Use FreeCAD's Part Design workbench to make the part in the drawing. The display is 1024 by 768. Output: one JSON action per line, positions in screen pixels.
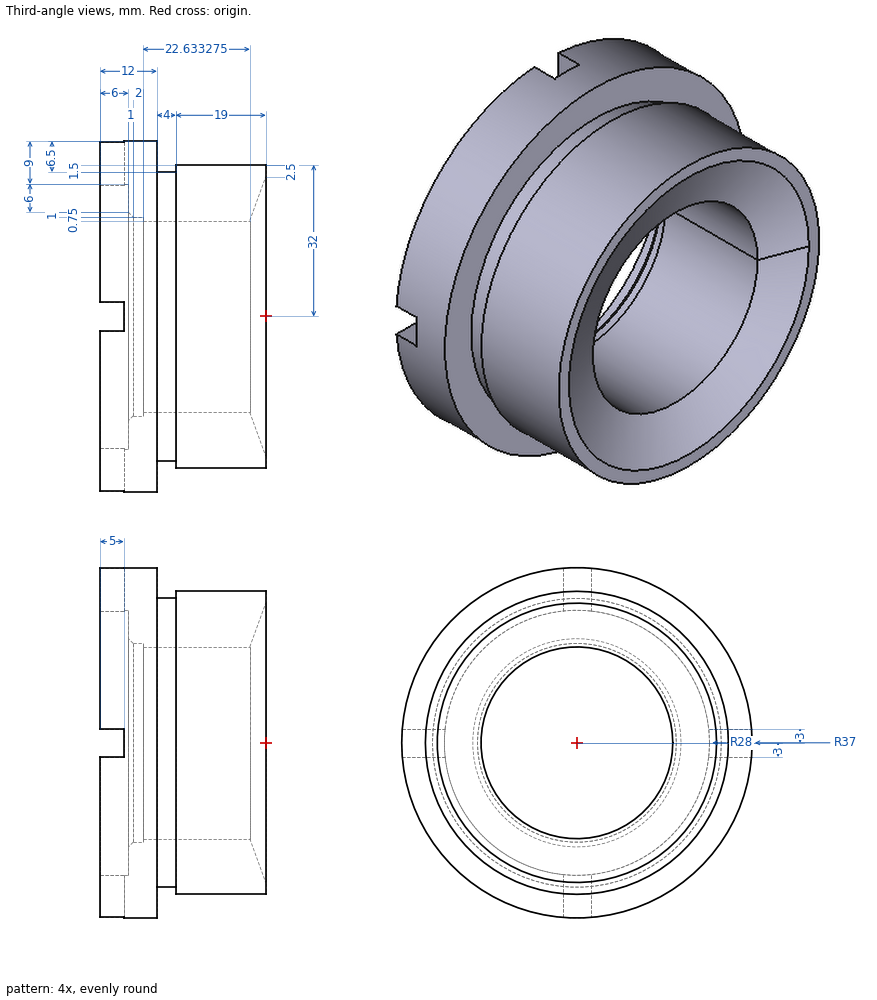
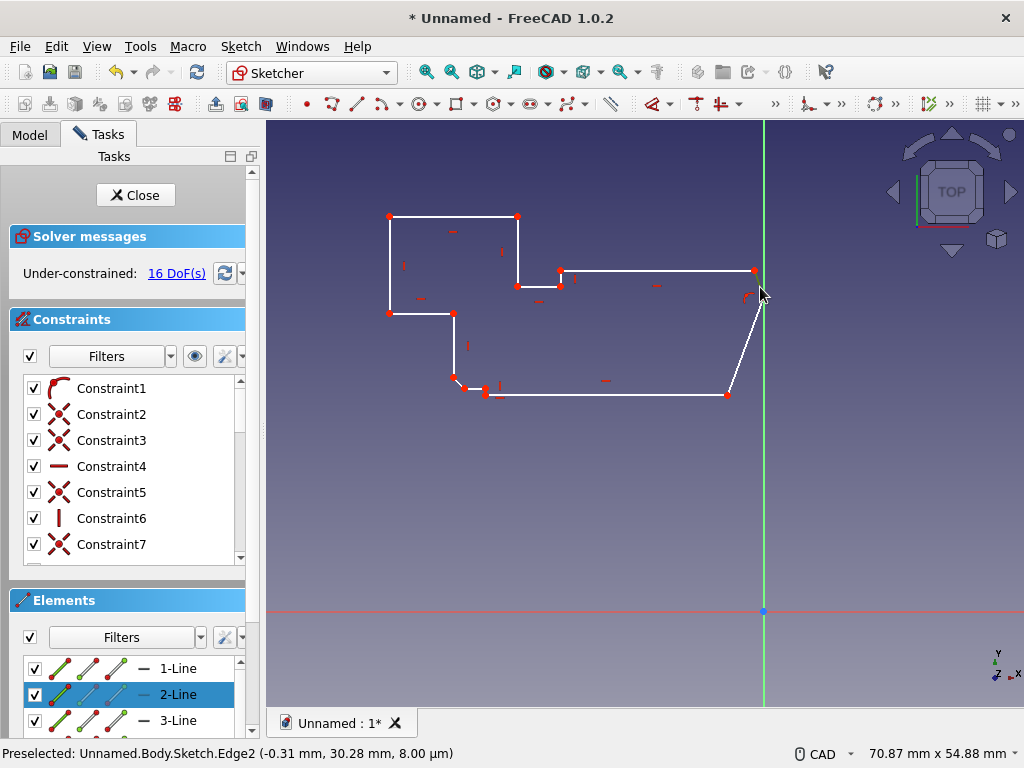
{"action": "left_click", "coordinate": [738, 104]}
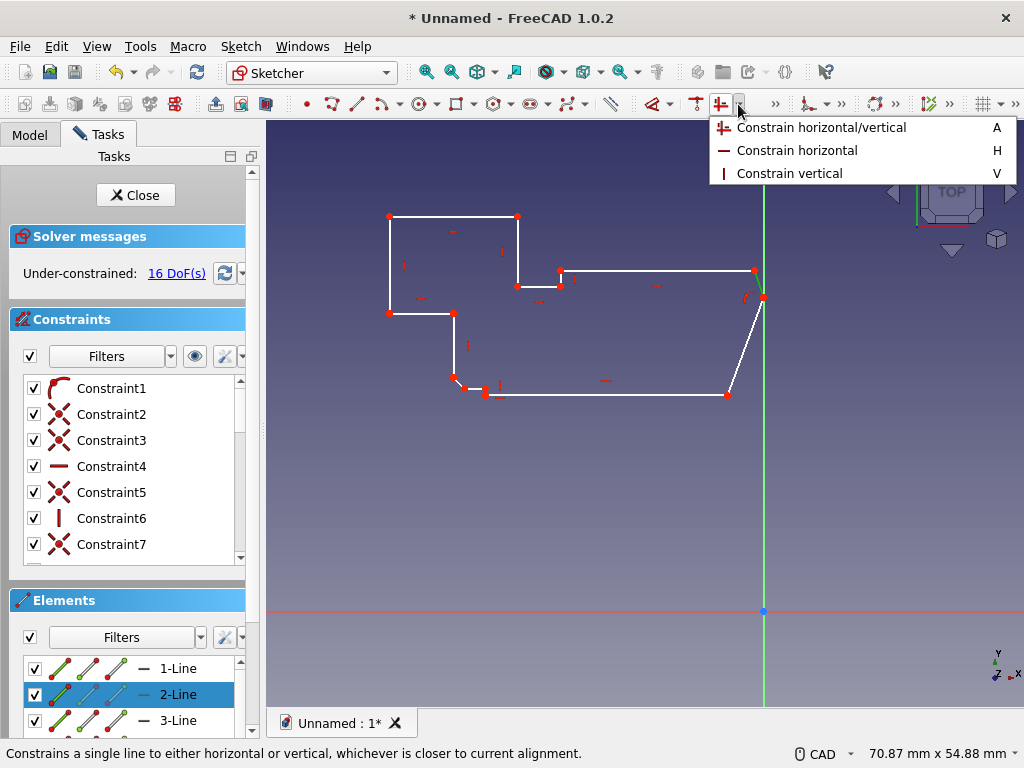
{"action": "left_click", "coordinate": [863, 174]}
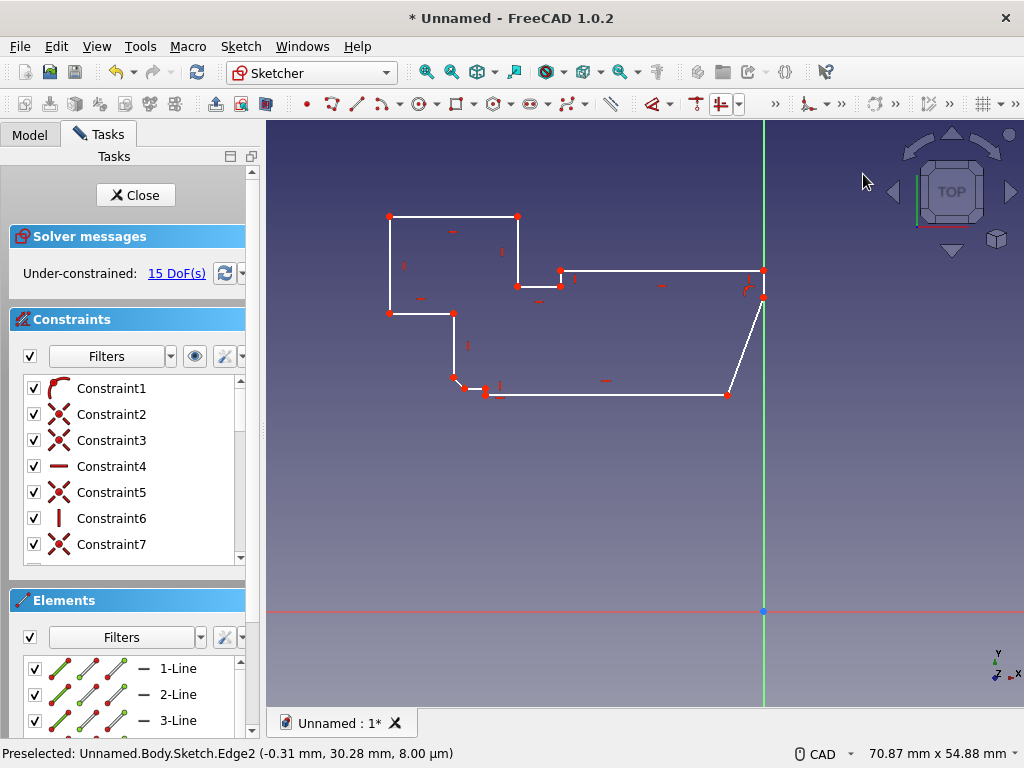
{"action": "left_click", "coordinate": [652, 104]}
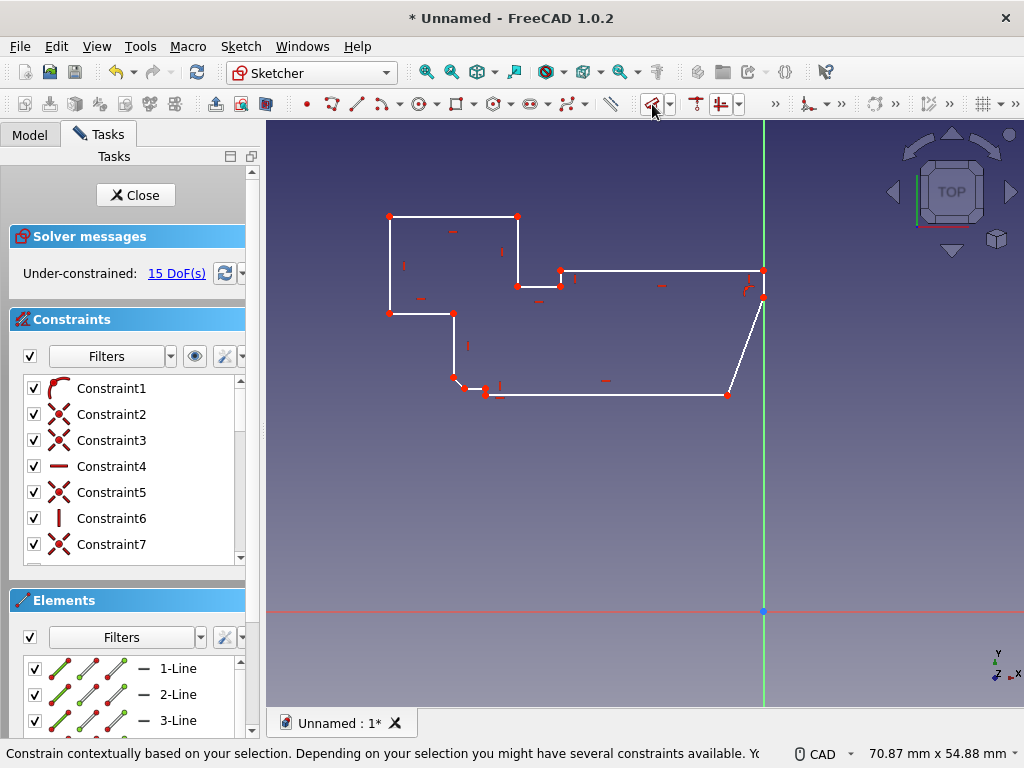
{"action": "left_click", "coordinate": [548, 287]}
{"action": "left_click", "coordinate": [539, 253]}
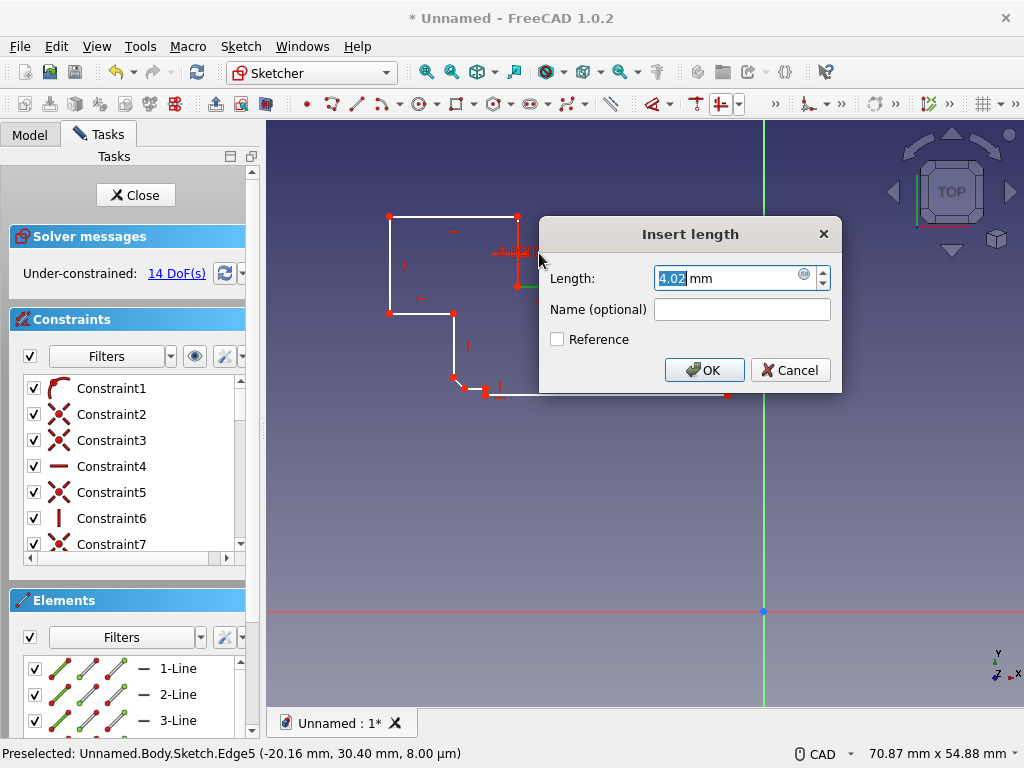
{"action": "type", "text": "4"}
{"action": "key", "text": "Return"}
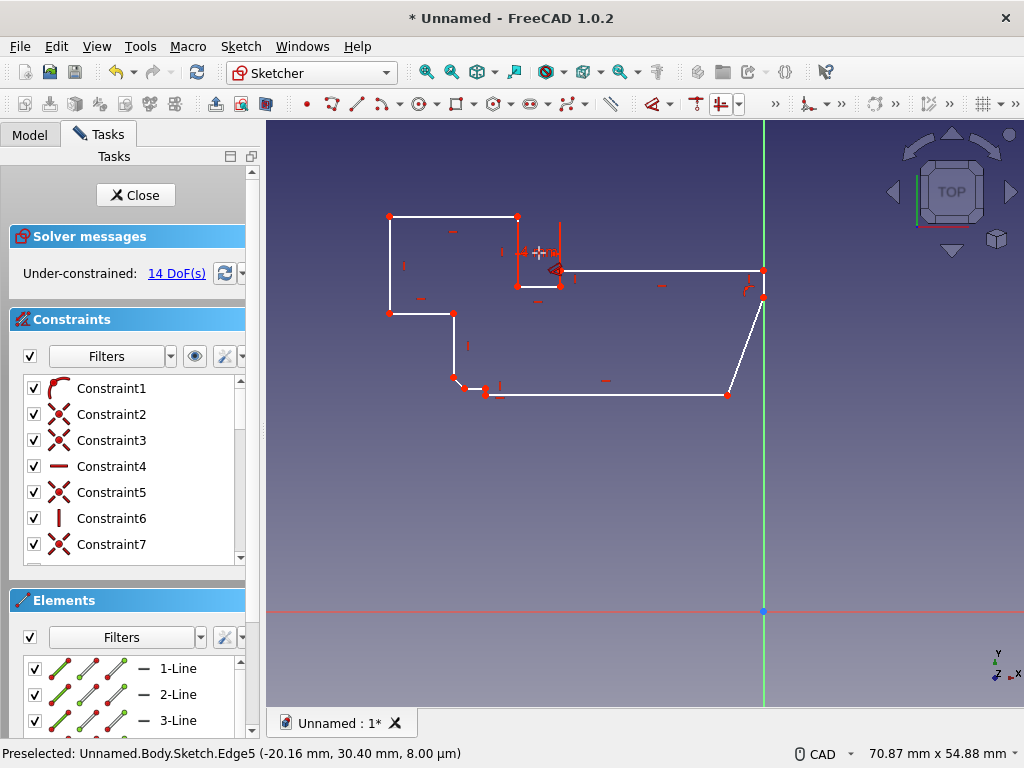
{"action": "left_click", "coordinate": [390, 246]}
{"action": "left_click", "coordinate": [356, 265]}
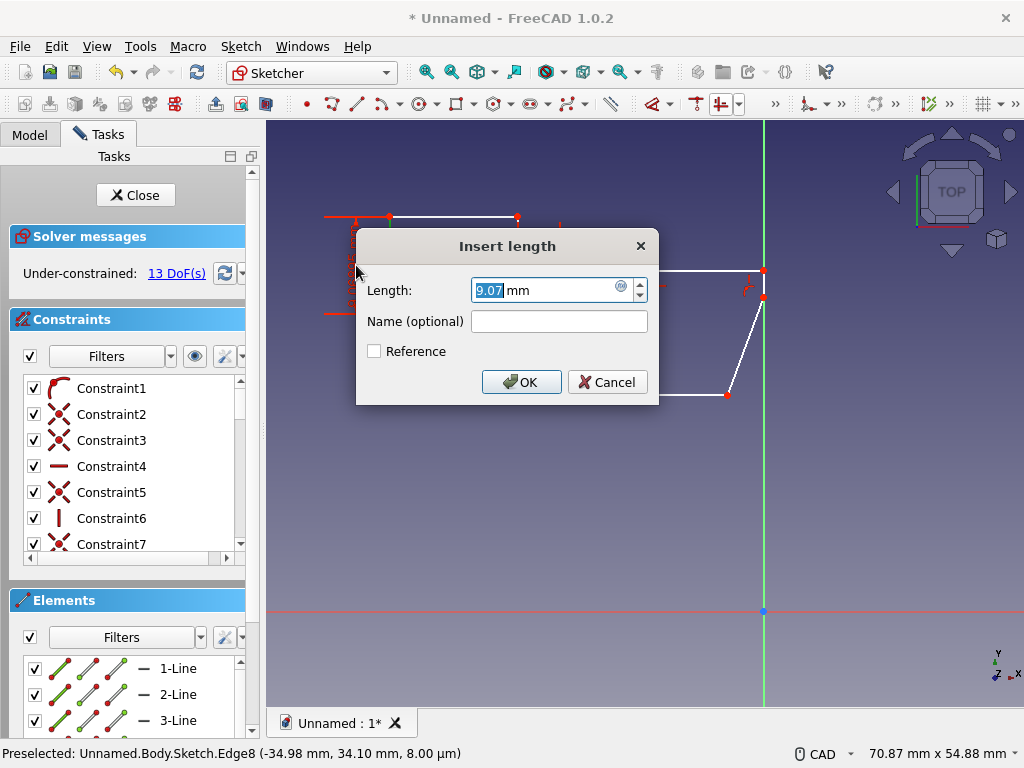
{"action": "type", "text": "9"}
{"action": "key", "text": "Return"}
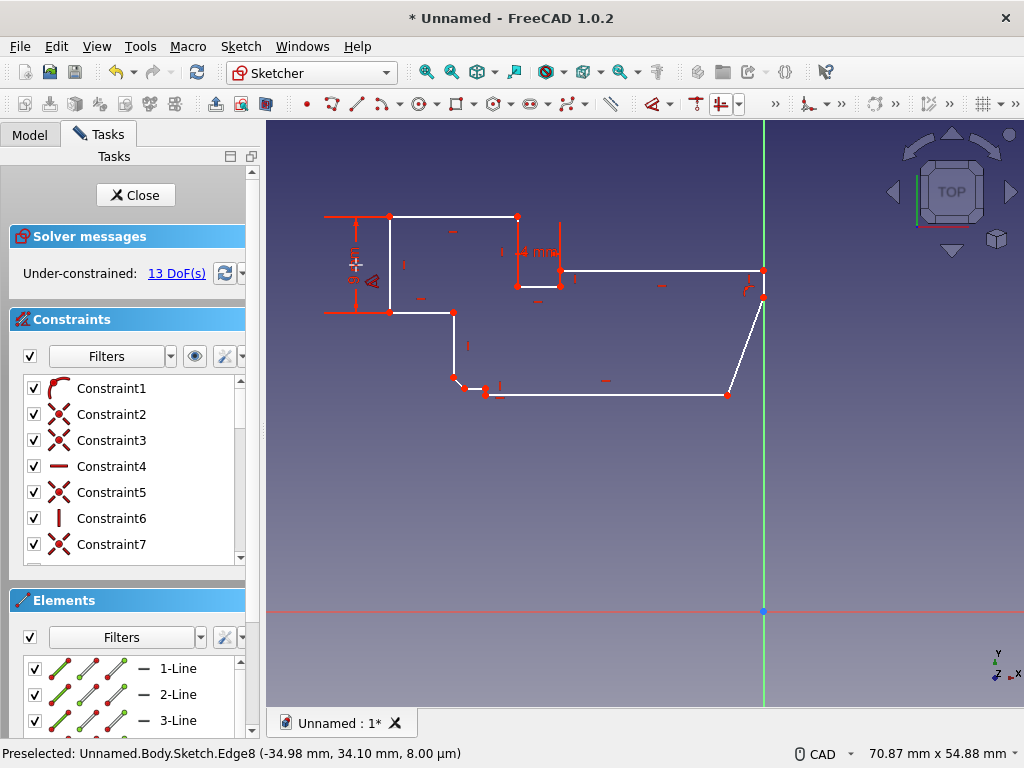
{"action": "left_click", "coordinate": [409, 313]}
{"action": "left_click", "coordinate": [436, 279]}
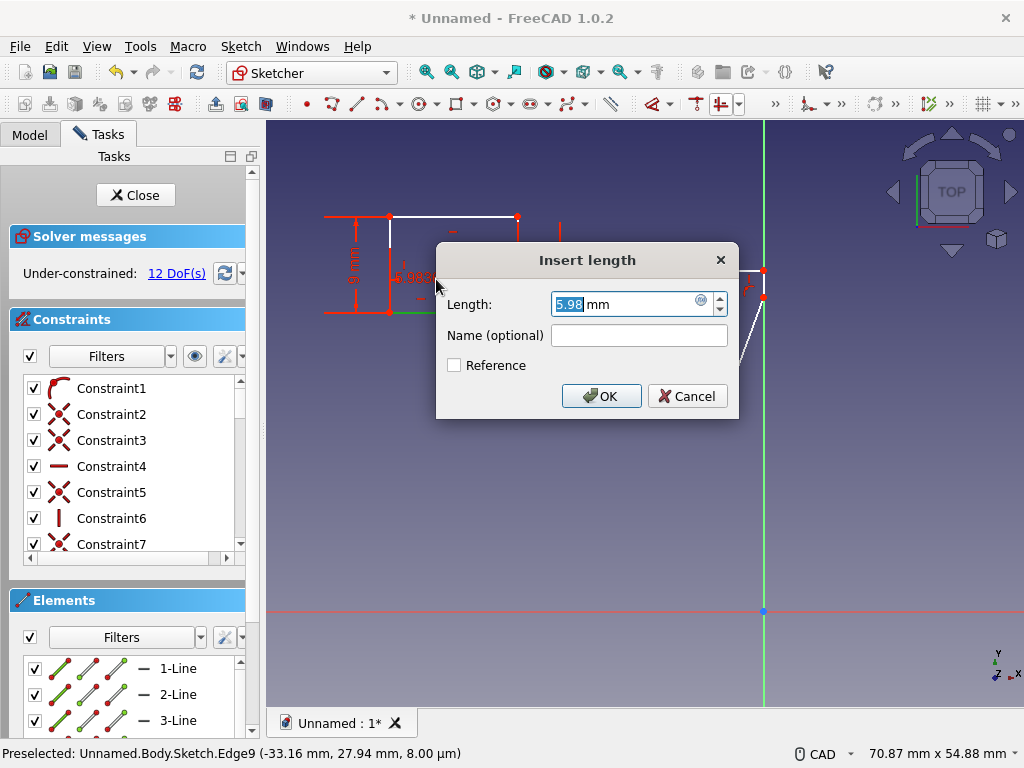
{"action": "type", "text": "6"}
{"action": "key", "text": "Return"}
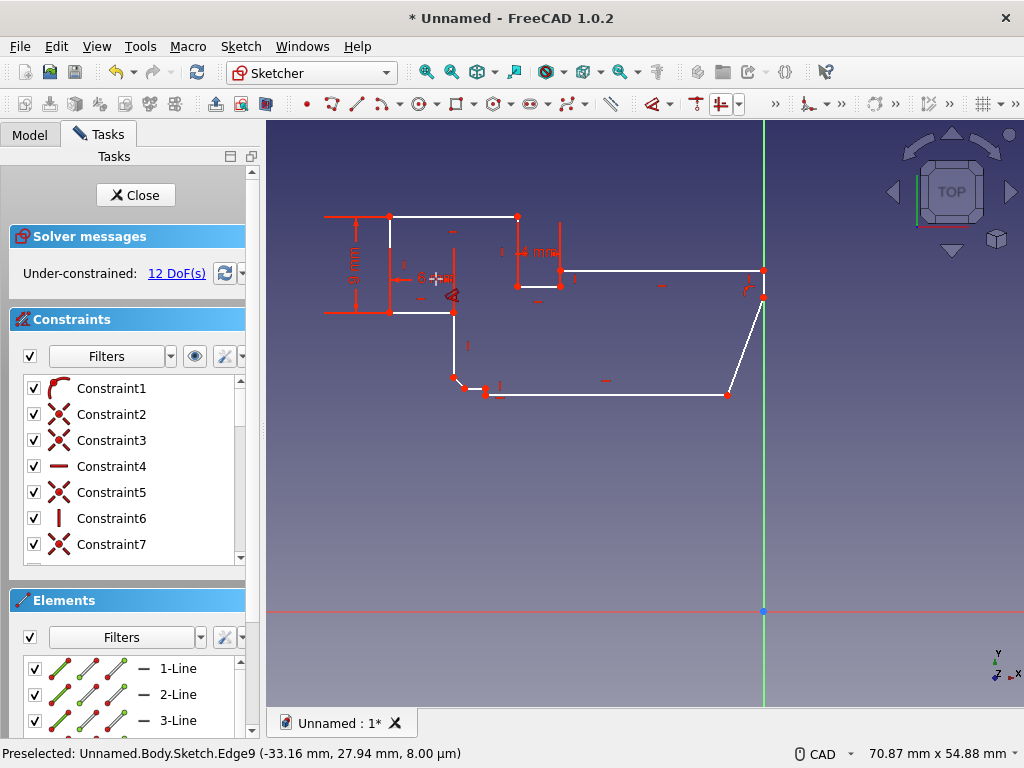
{"action": "left_click", "coordinate": [454, 332]}
{"action": "left_click", "coordinate": [420, 345]}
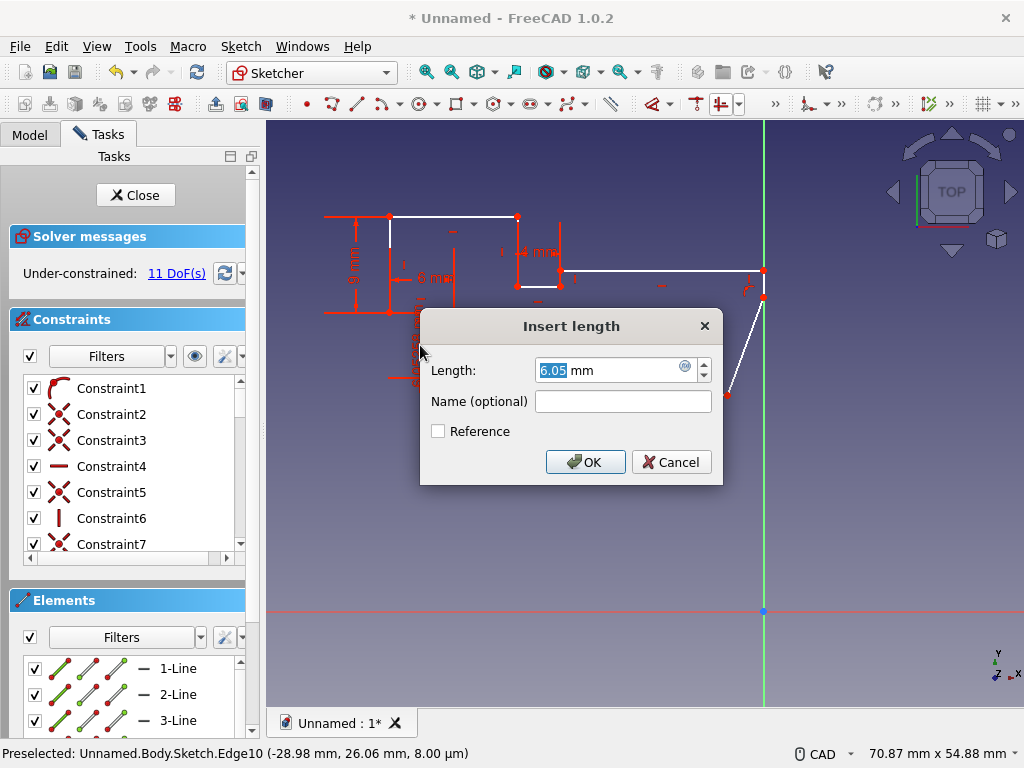
{"action": "type", "text": "6"}
{"action": "key", "text": "Return"}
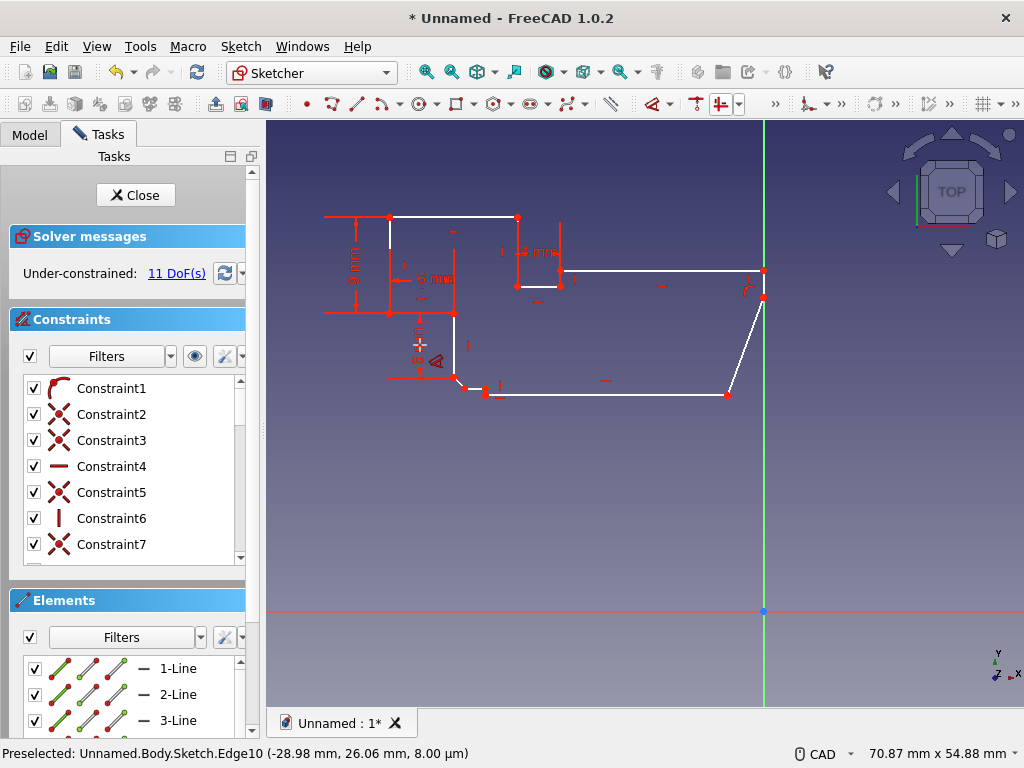
{"action": "scroll", "coordinate": [475, 389], "scroll_direction": "up", "scroll_amount": 4}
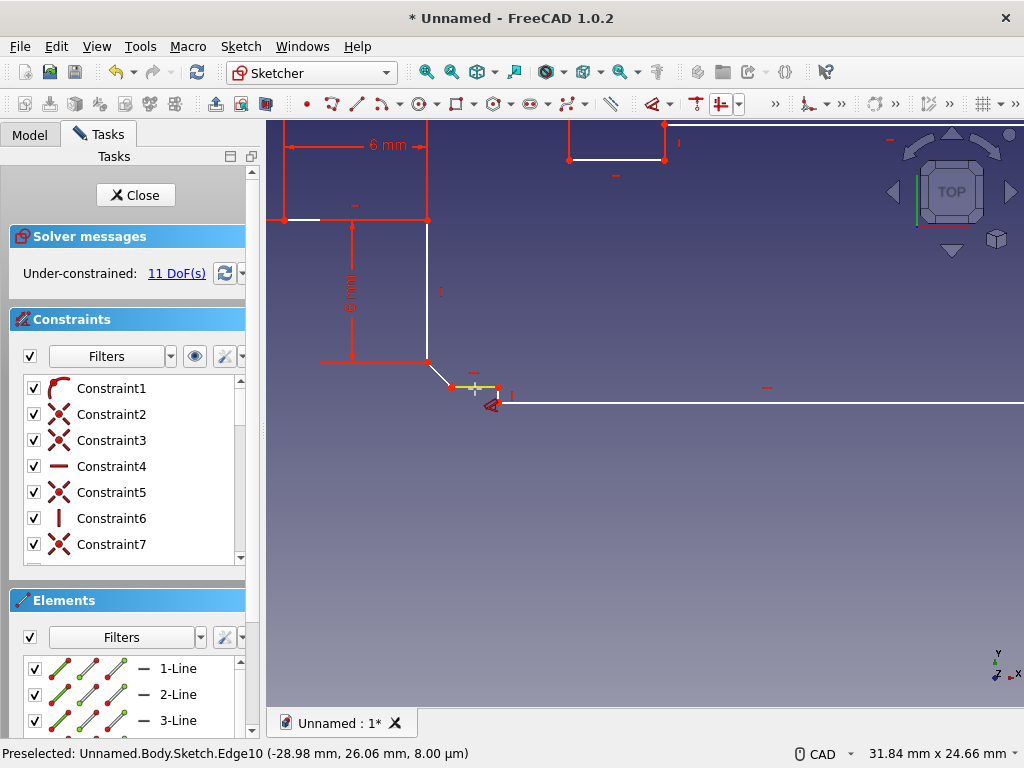
{"action": "left_click", "coordinate": [475, 387]}
{"action": "left_click", "coordinate": [475, 353]}